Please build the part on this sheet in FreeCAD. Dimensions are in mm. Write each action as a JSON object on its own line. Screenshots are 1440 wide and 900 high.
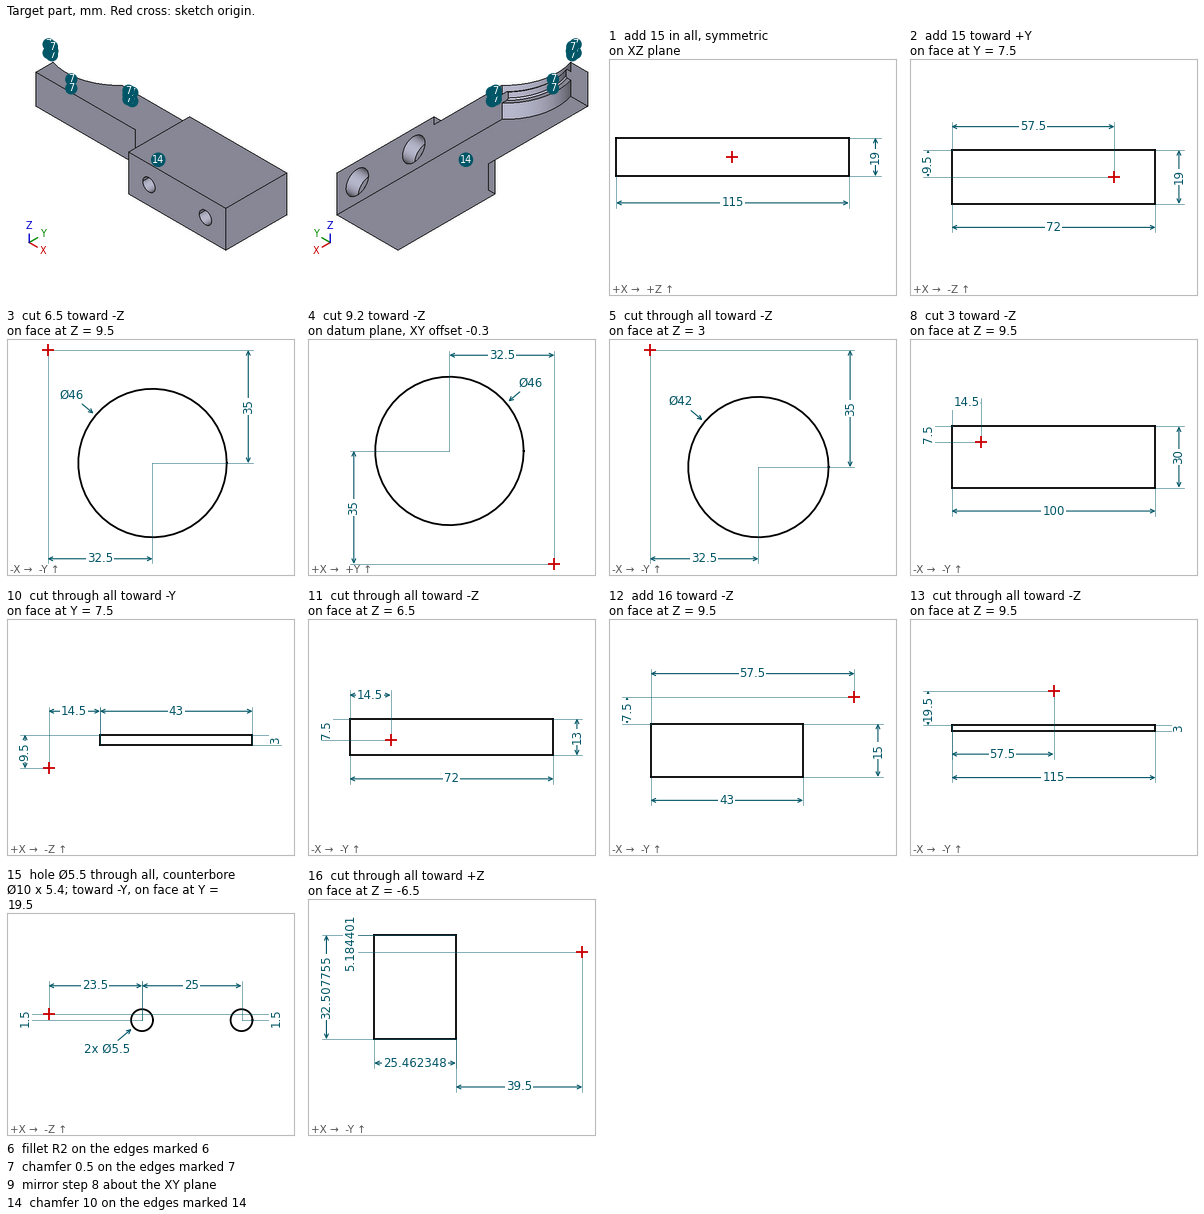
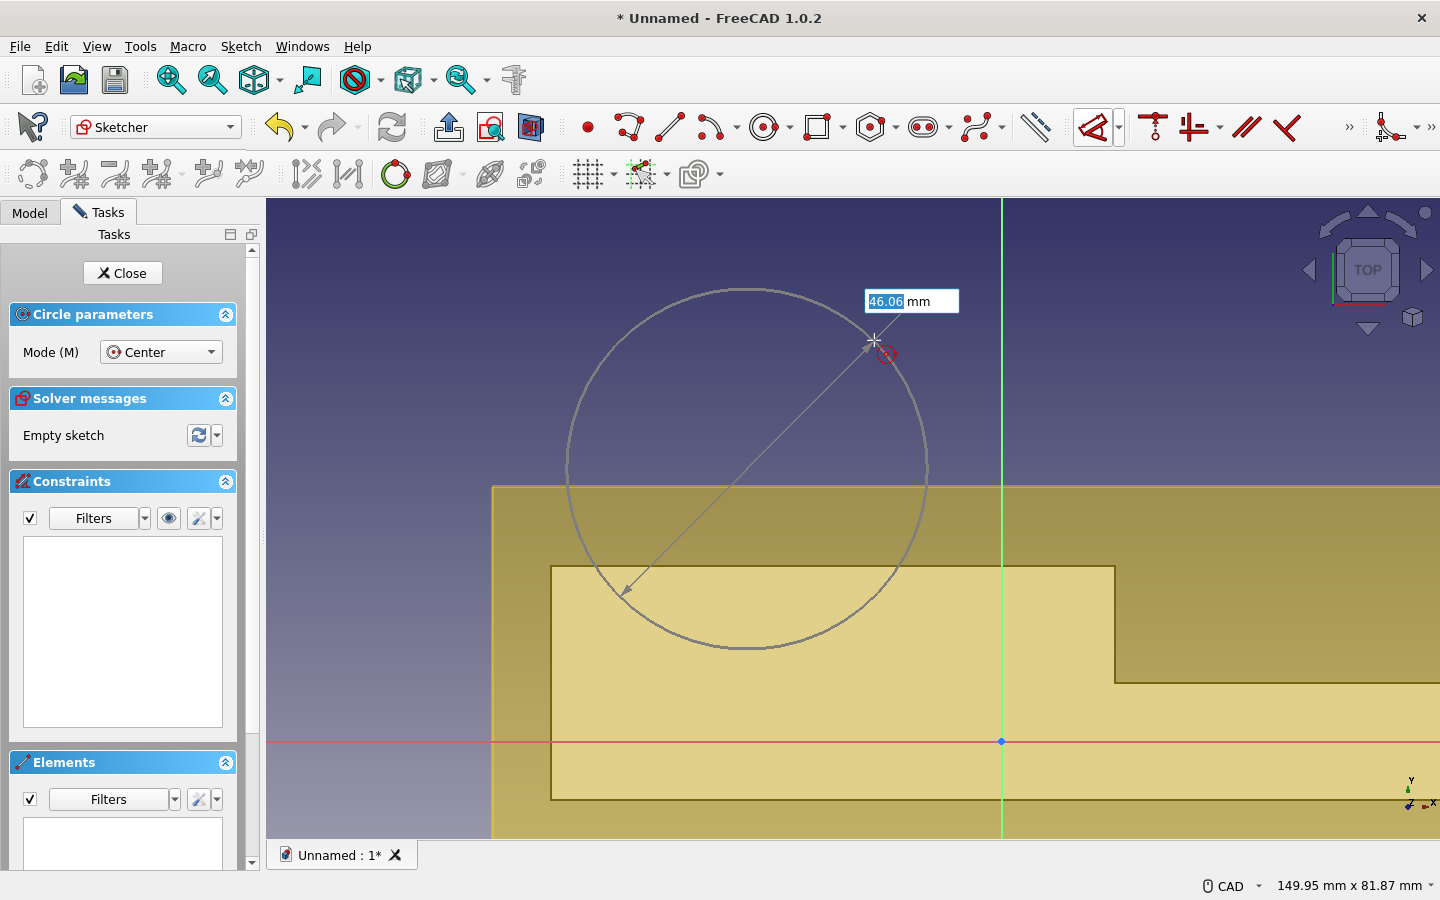
{"action": "type", "text": "46"}
{"action": "key", "text": "Return"}
{"action": "key", "text": "Escape"}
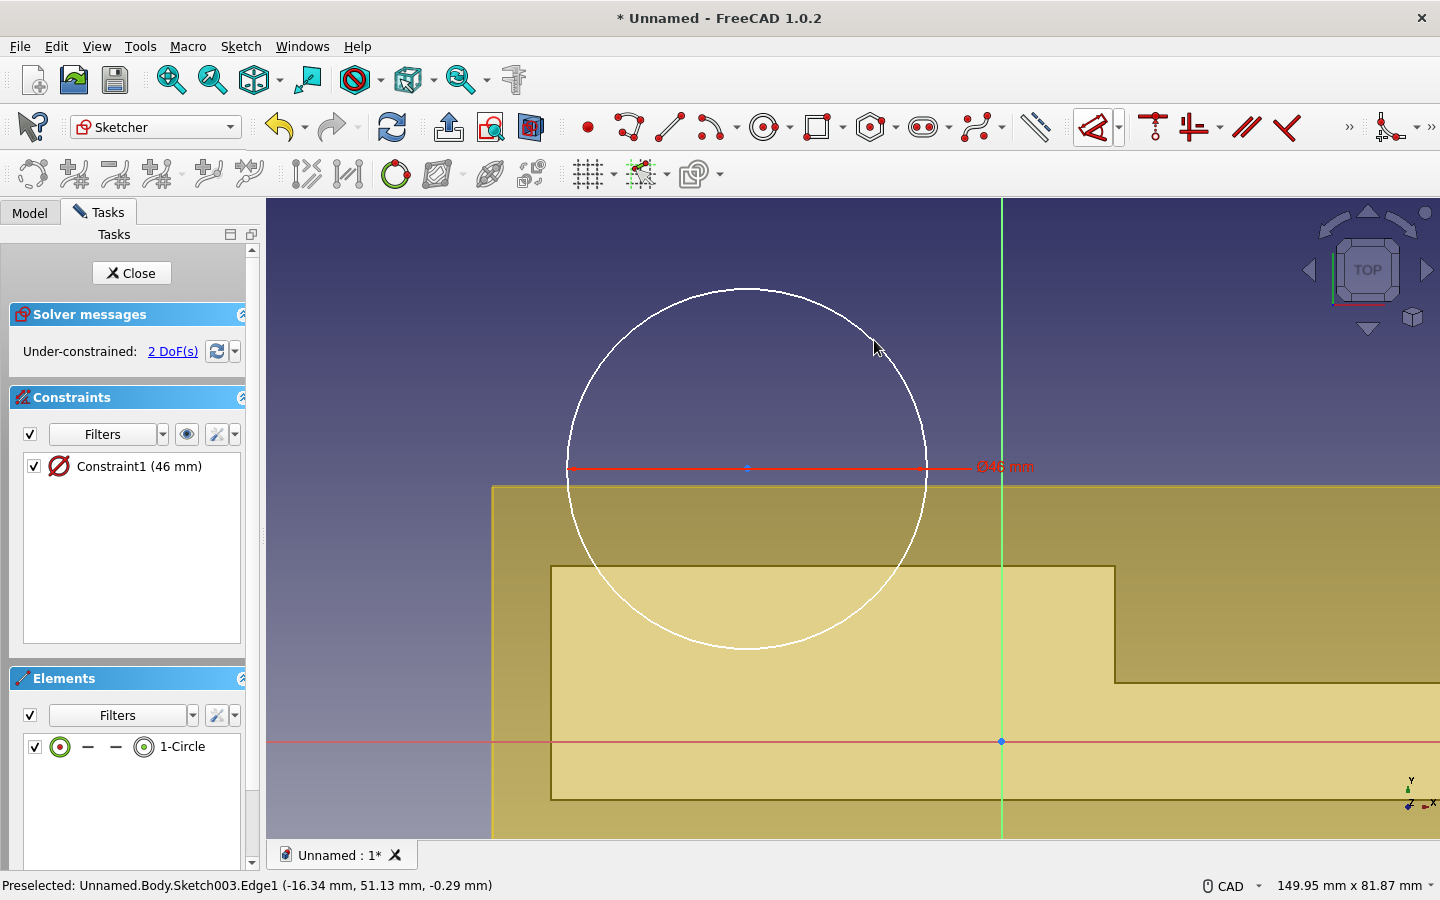
{"action": "left_click", "coordinate": [747, 469]}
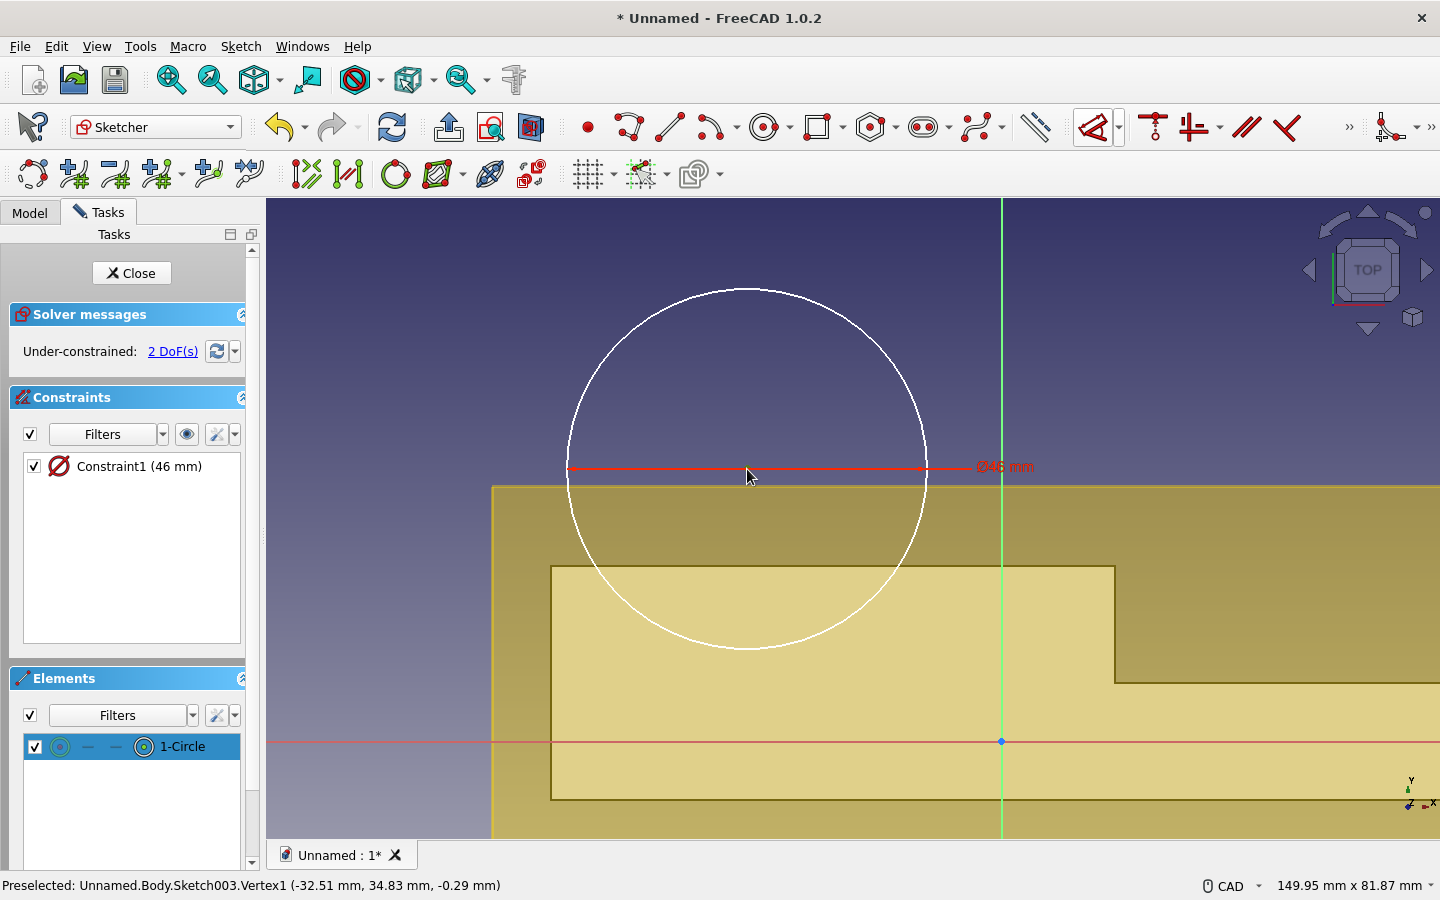
{"action": "left_click", "coordinate": [1118, 128]}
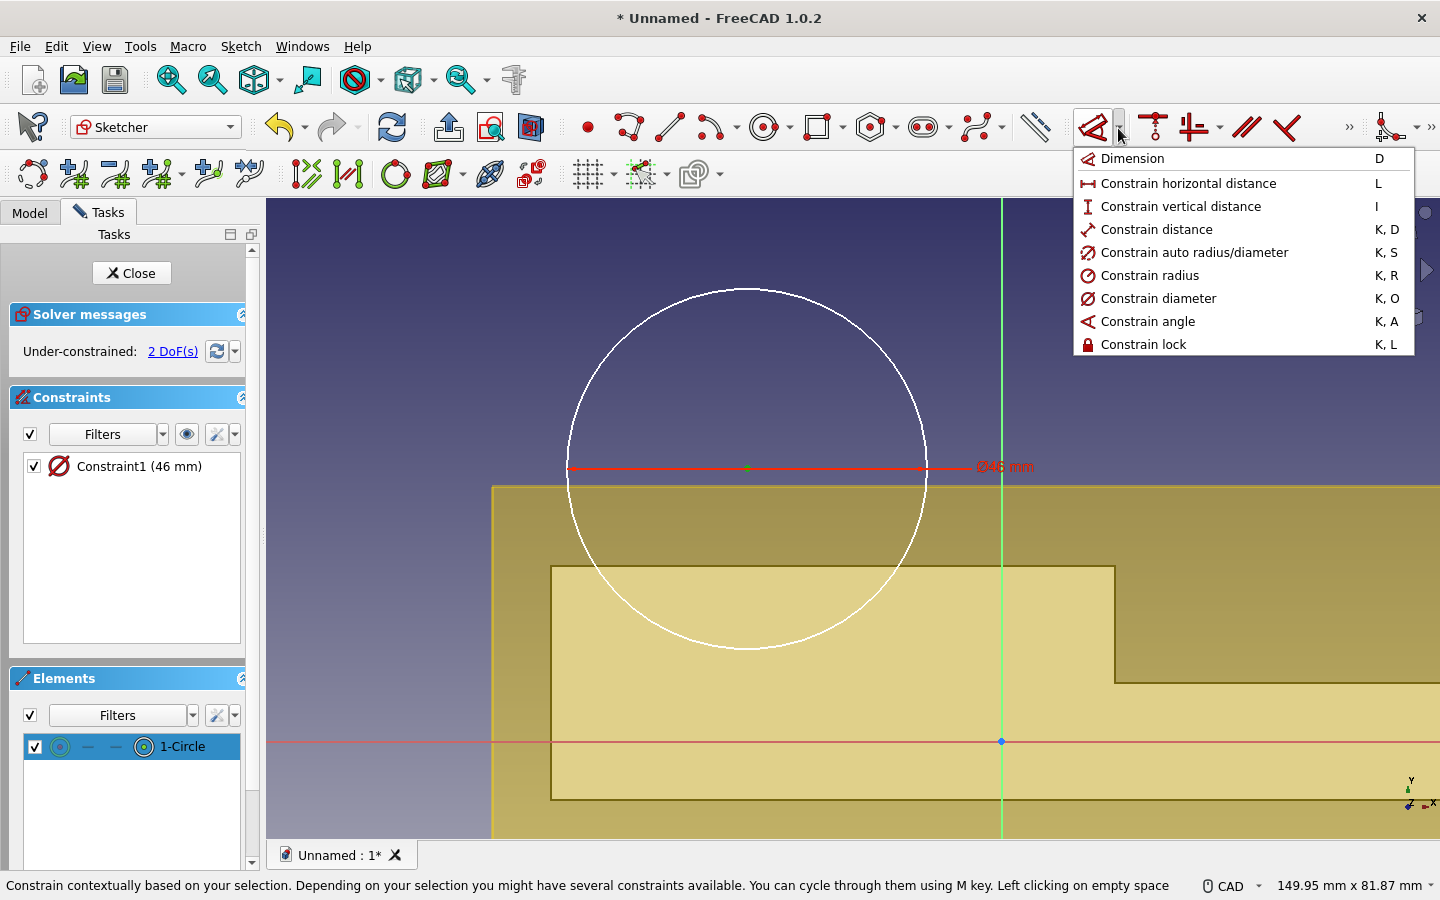
{"action": "left_click", "coordinate": [1244, 206]}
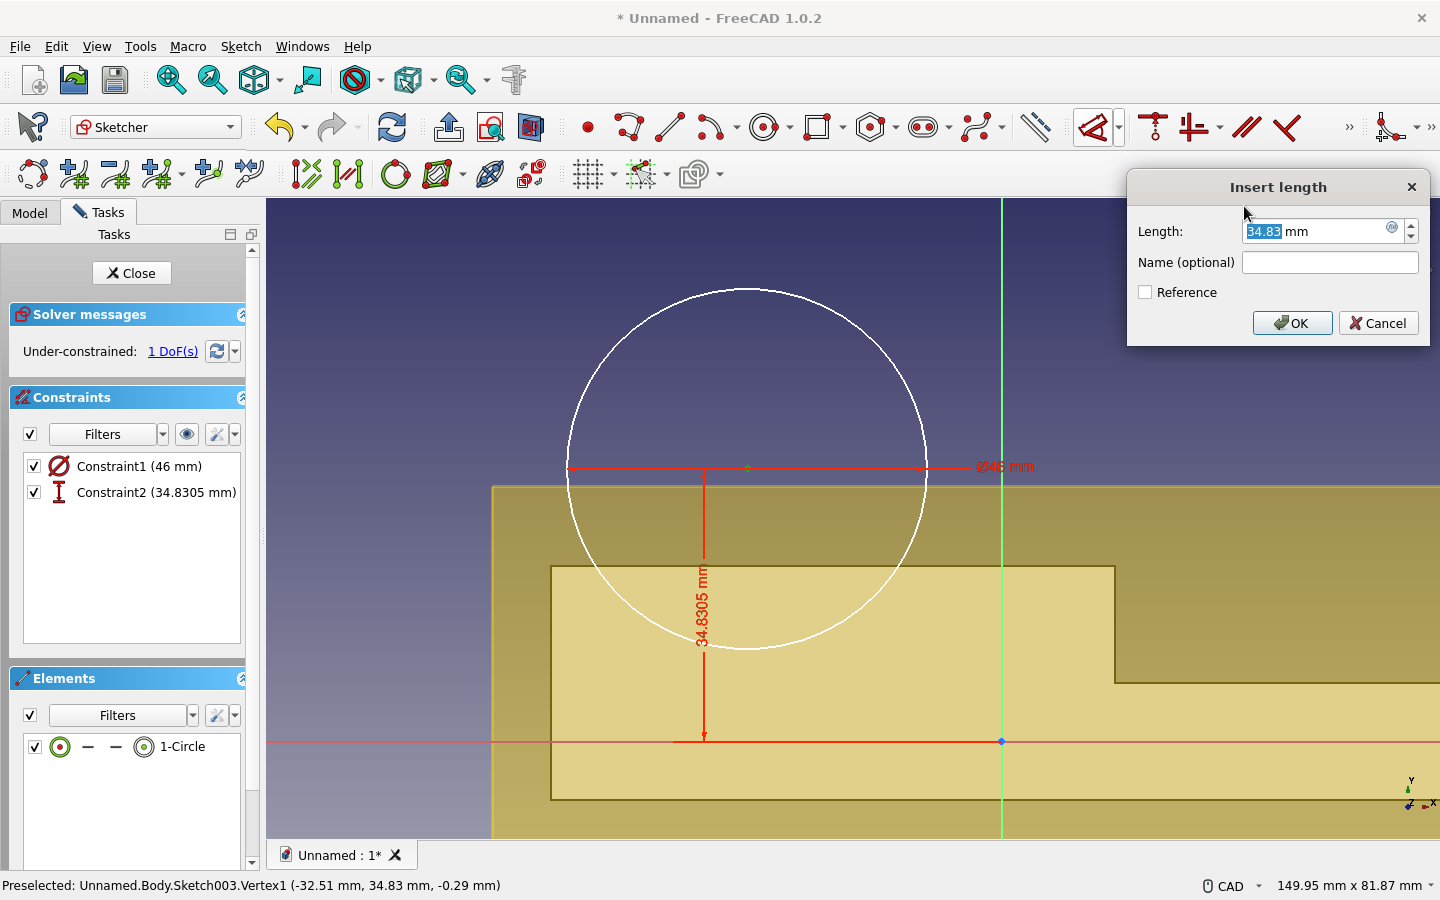
{"action": "type", "text": "35"}
{"action": "key", "text": "Return"}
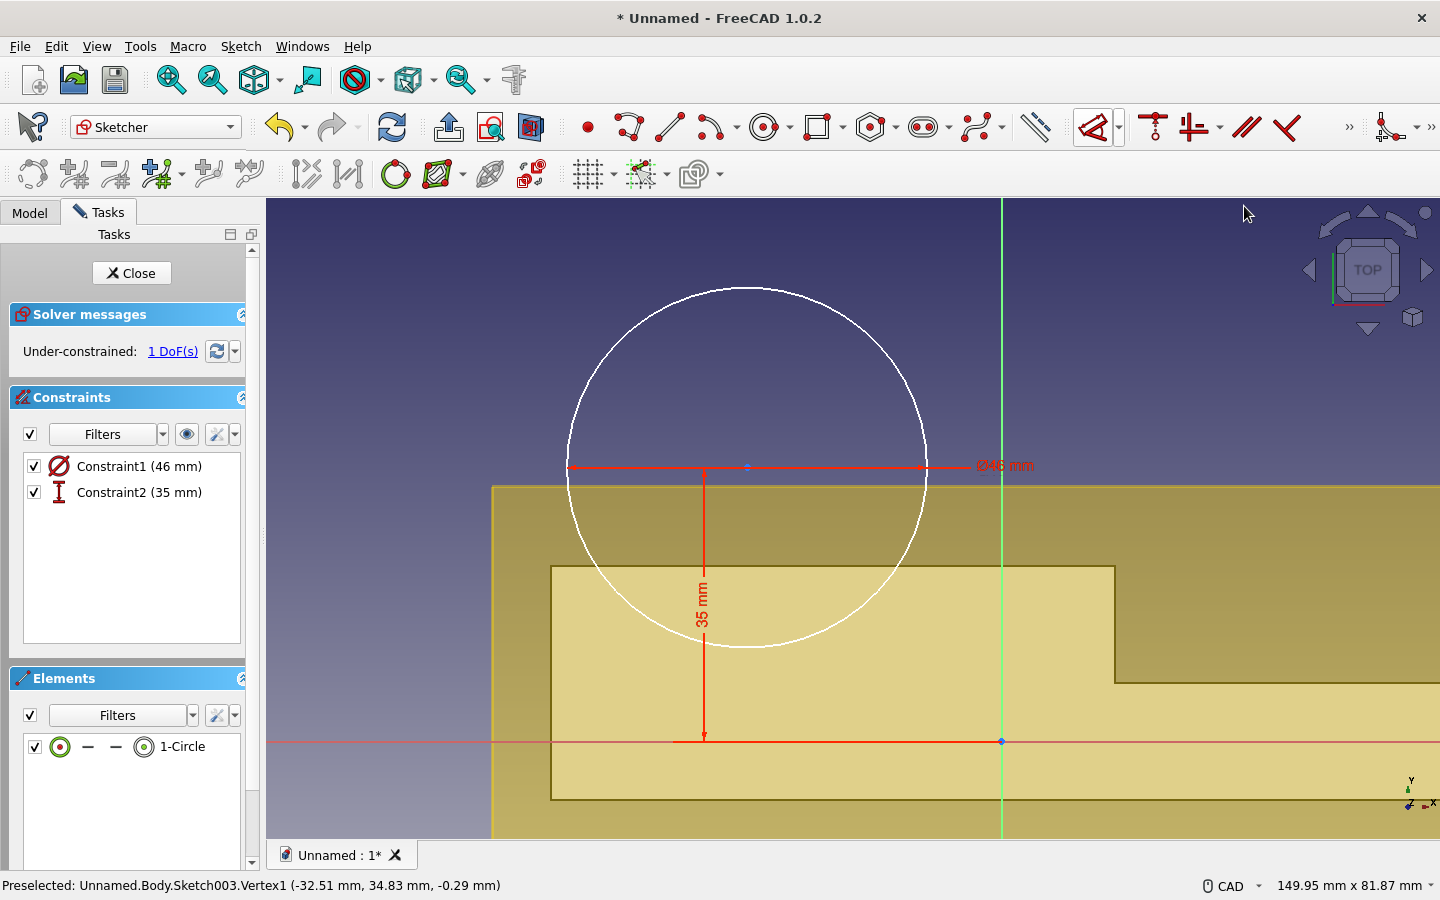
{"action": "left_click", "coordinate": [747, 468]}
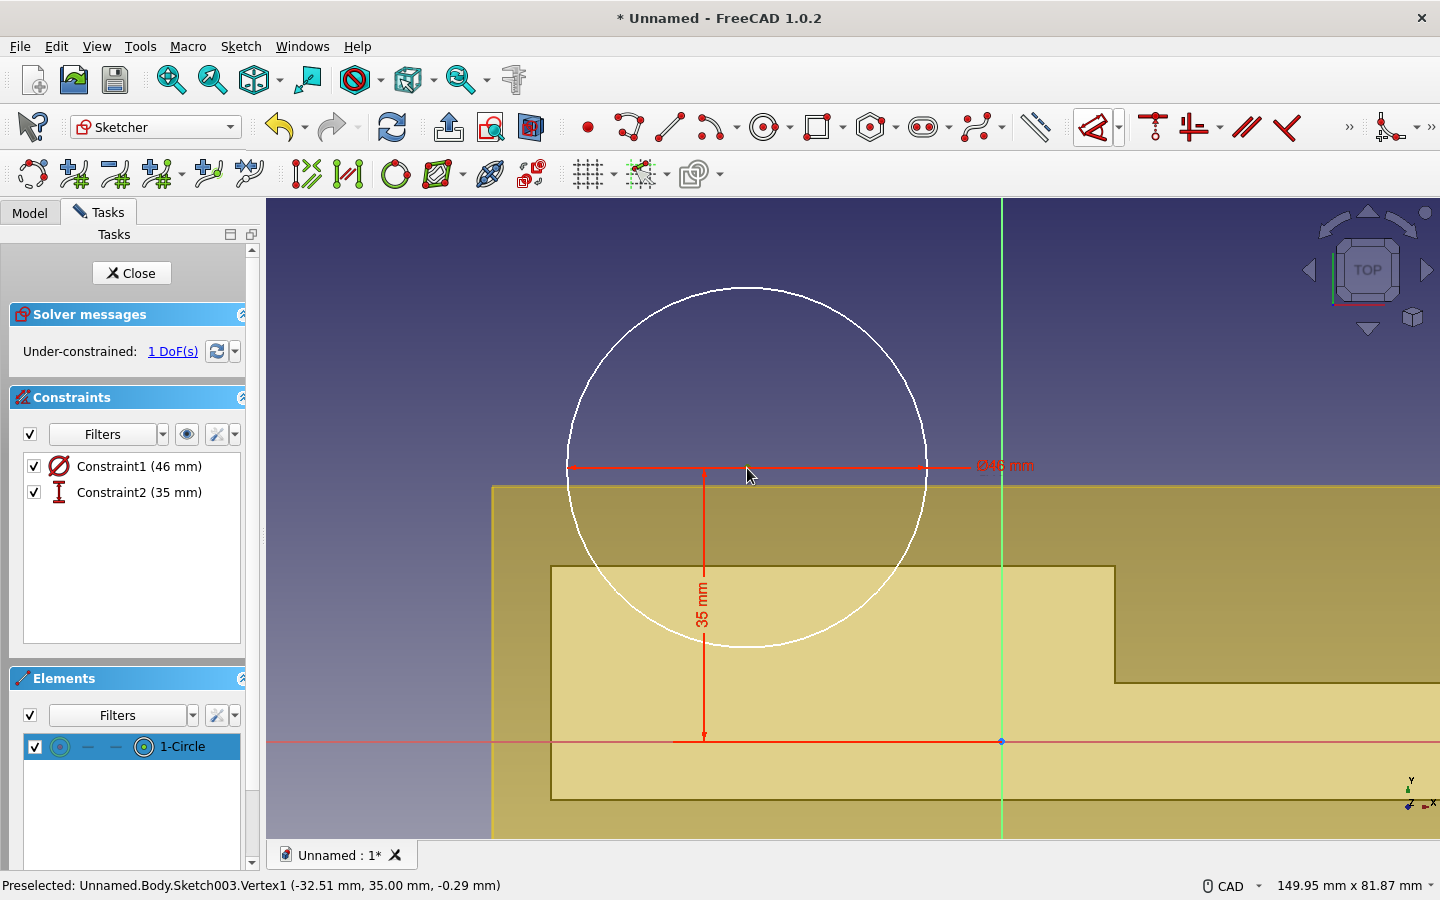
{"action": "key", "text": "l"}